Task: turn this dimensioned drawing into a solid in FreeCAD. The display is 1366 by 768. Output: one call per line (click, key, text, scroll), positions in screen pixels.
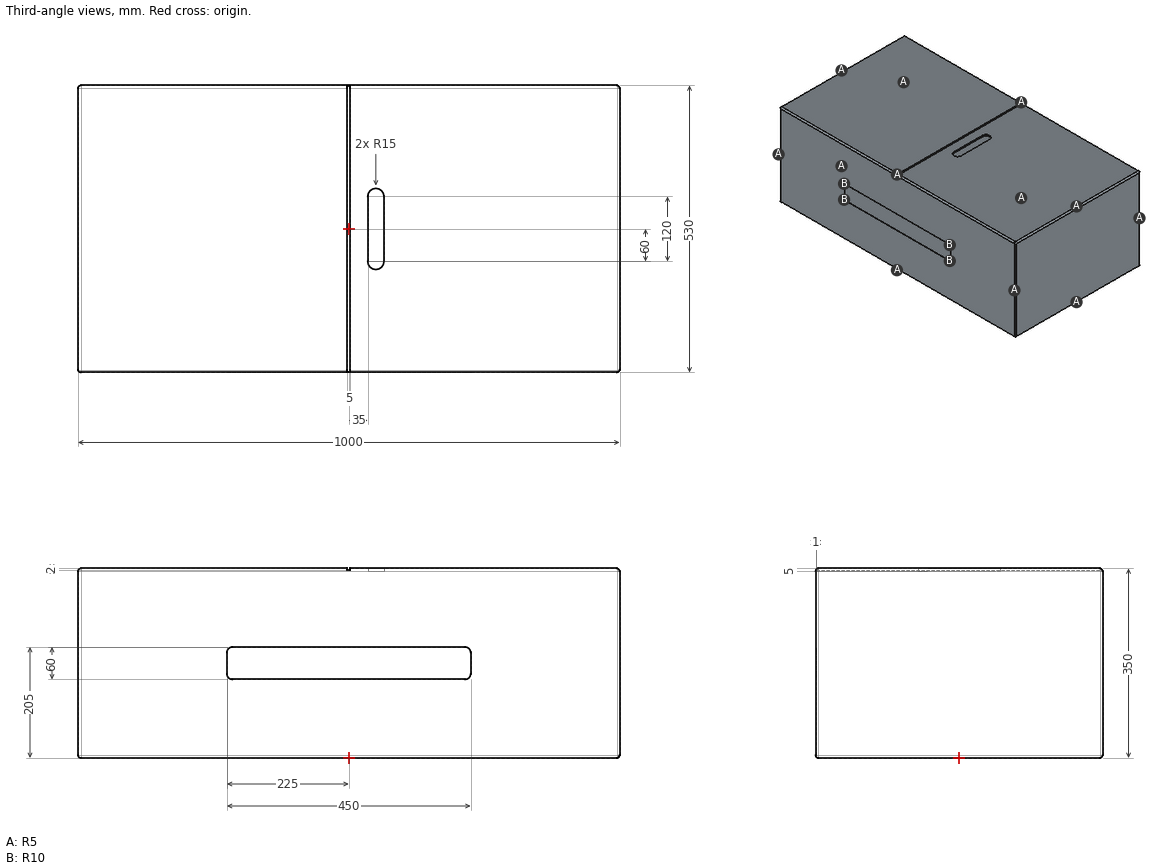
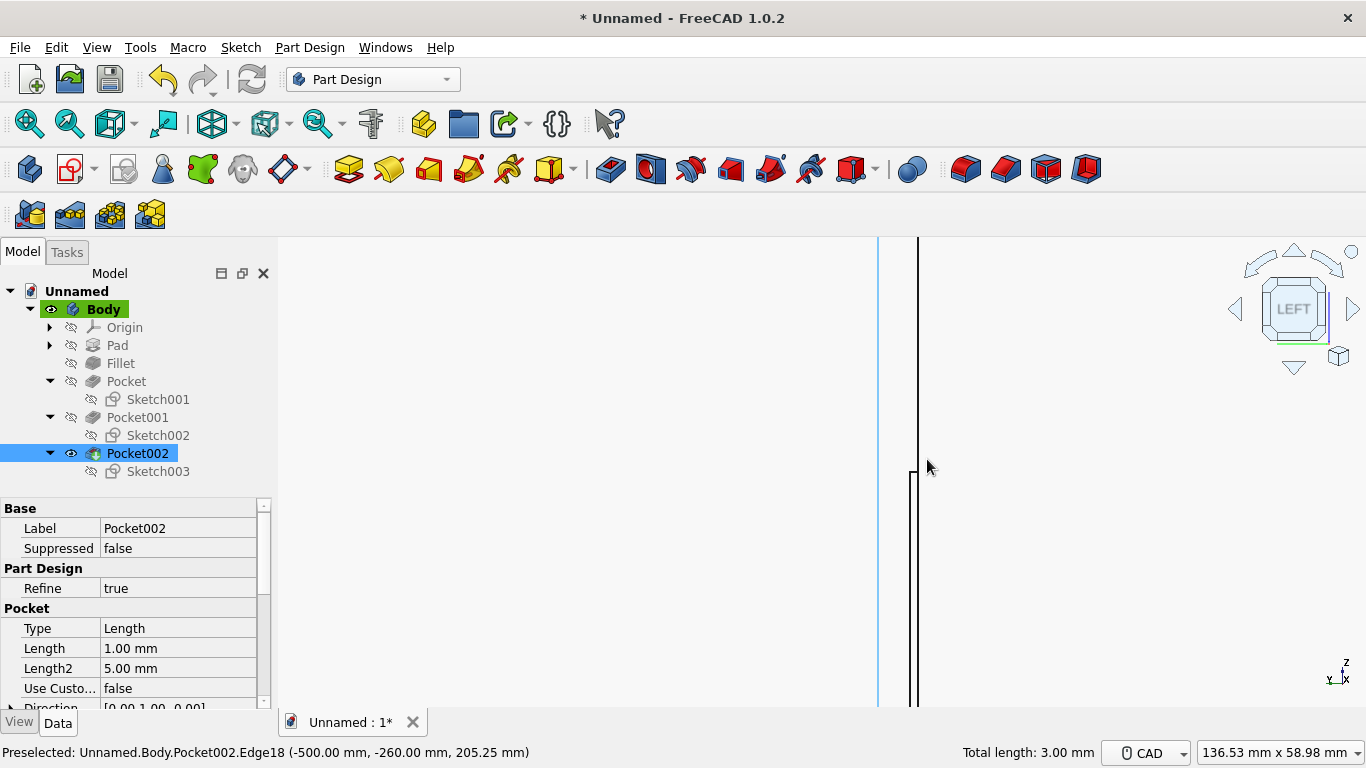
scroll(914, 471, up, 9)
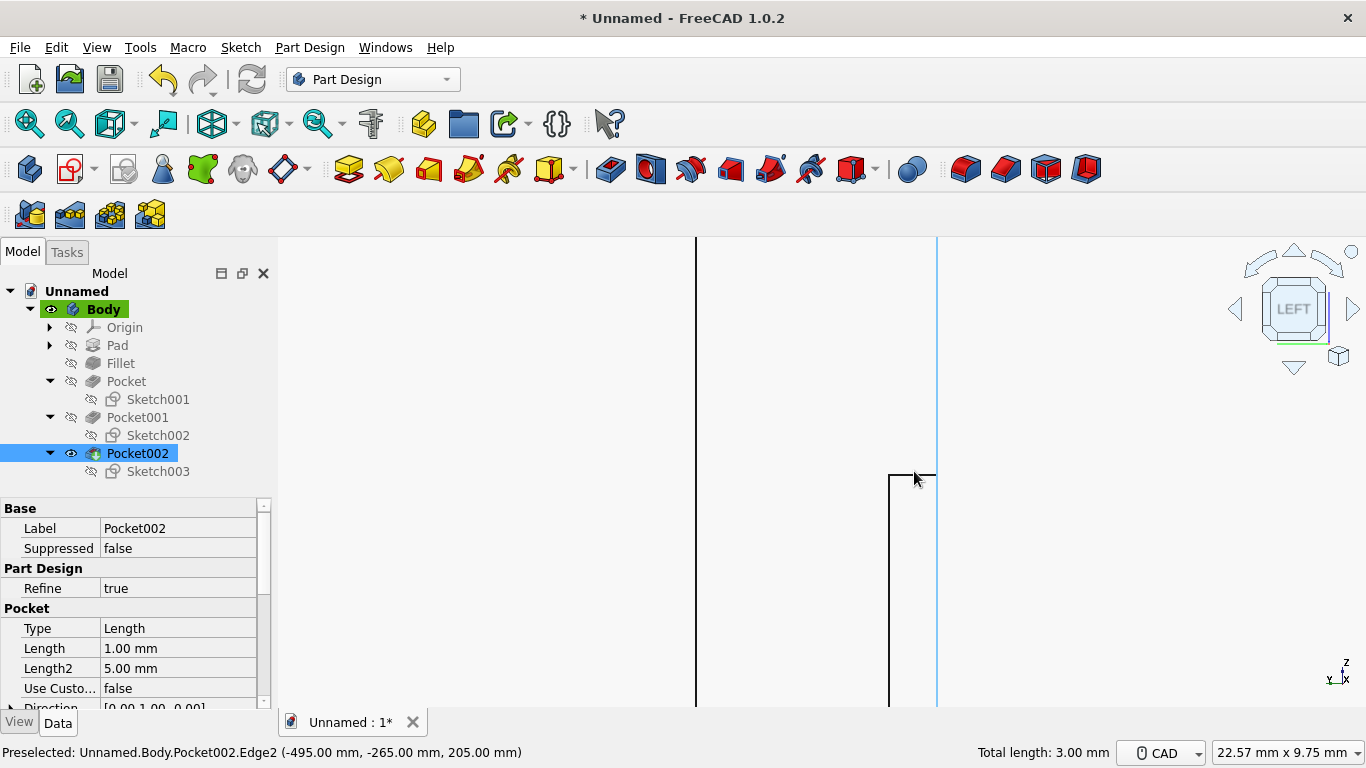
click(913, 474, ctrl)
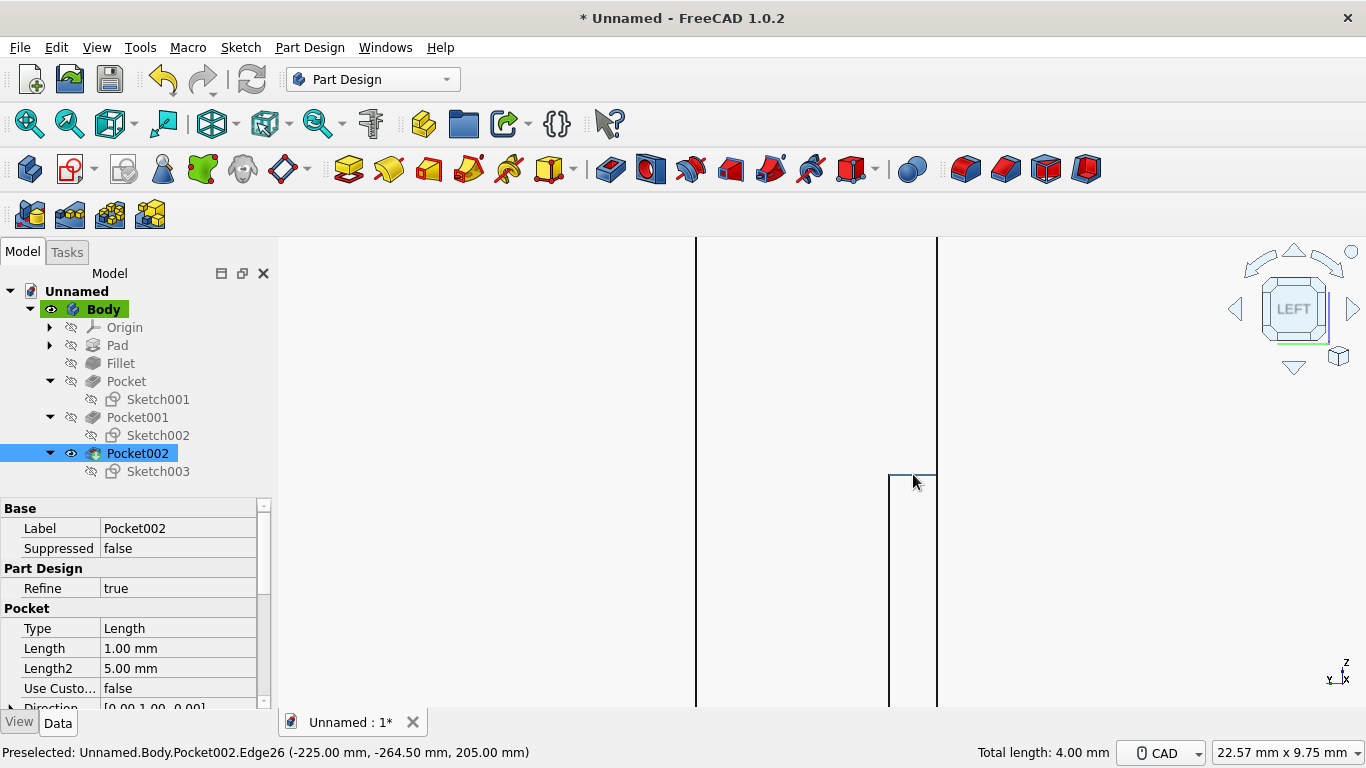
key(v)
key(1)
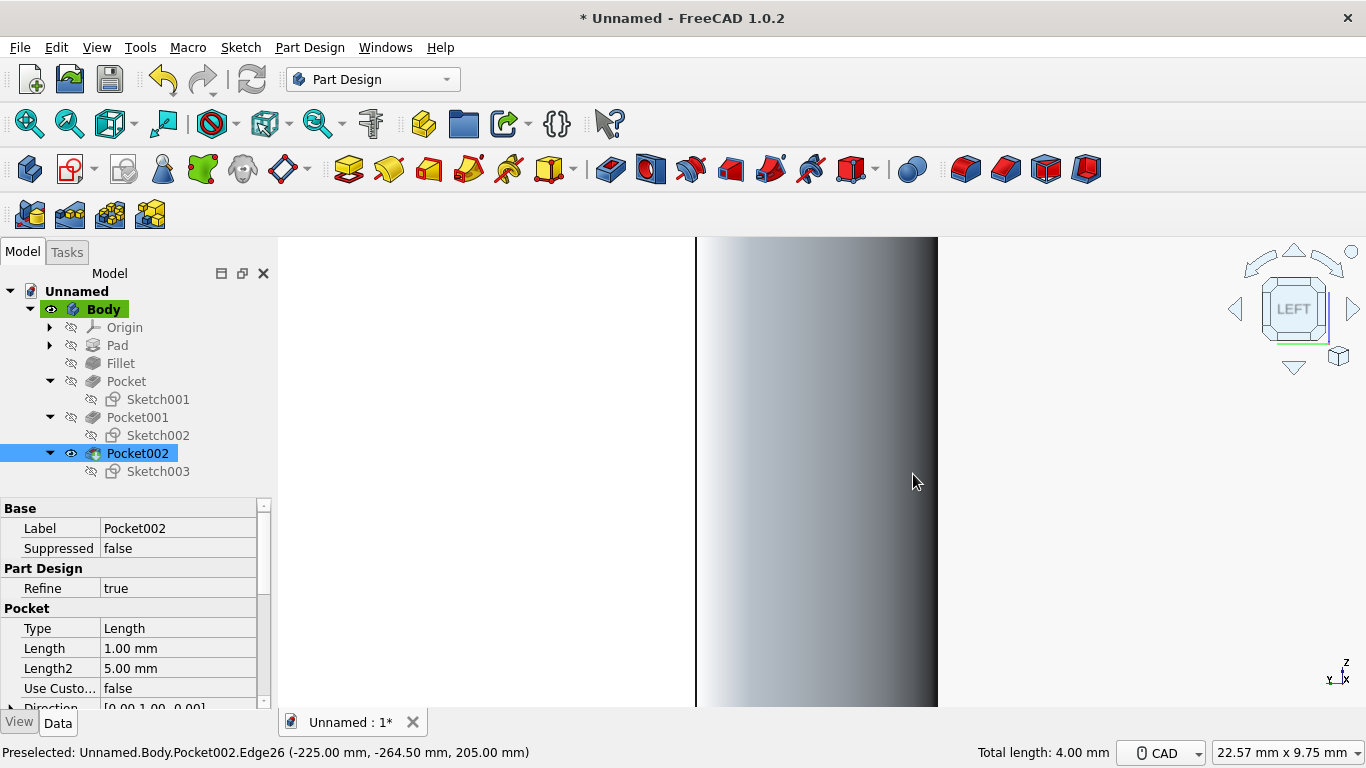
click(966, 170)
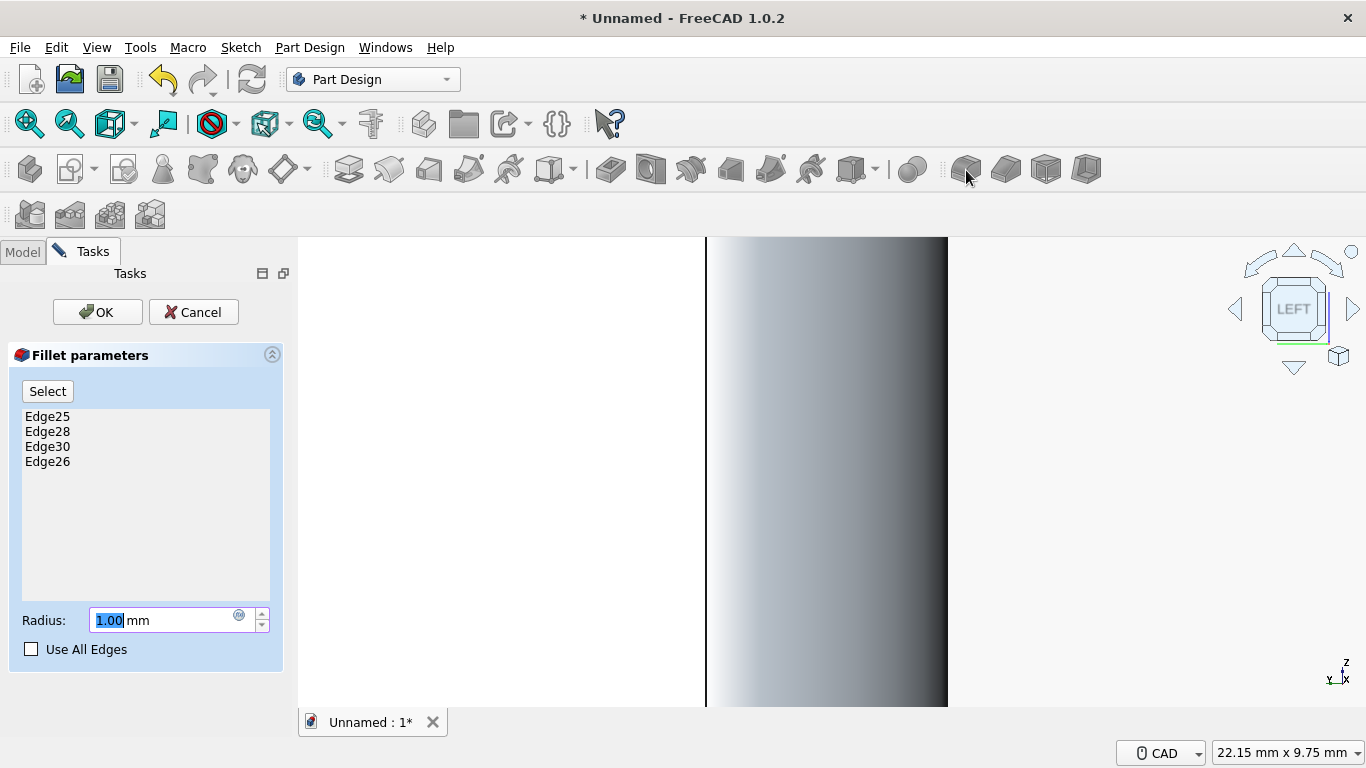
text(10)
key(Tab)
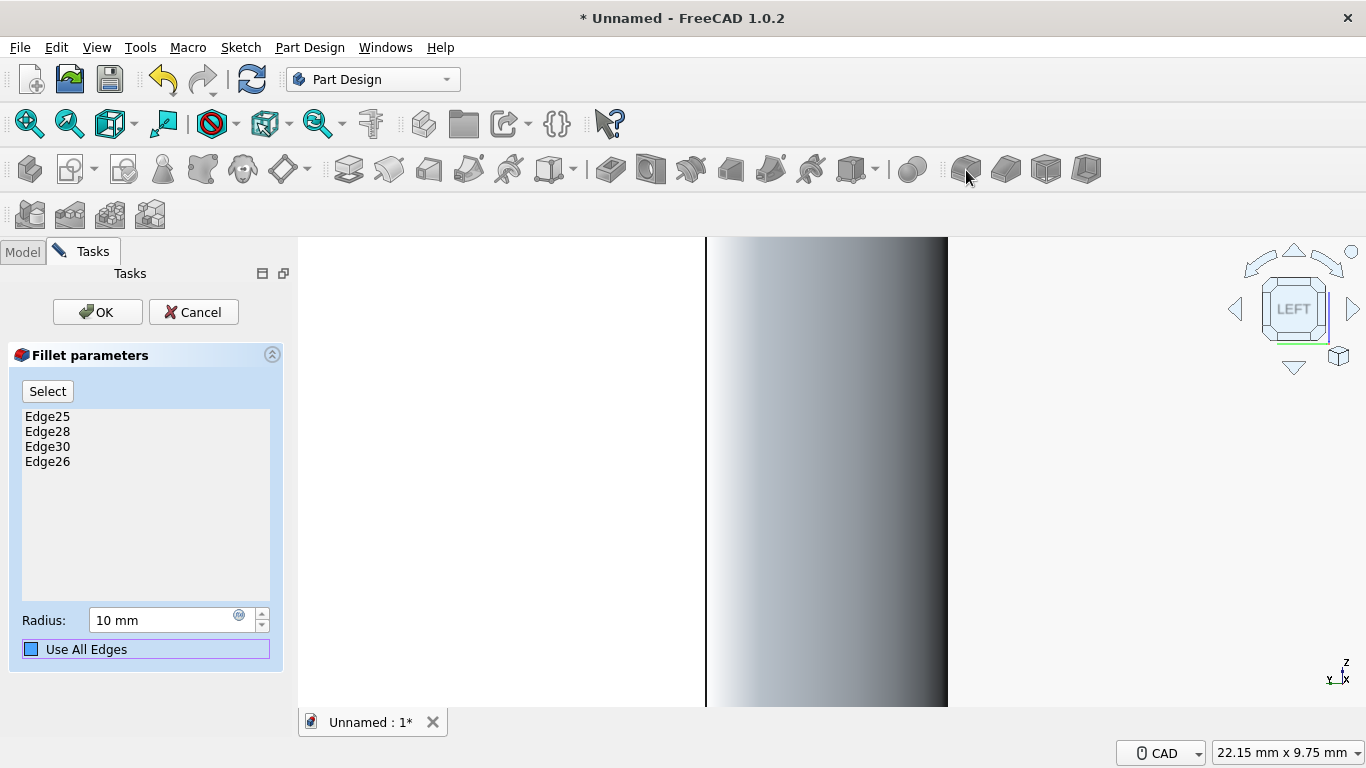
click(98, 312)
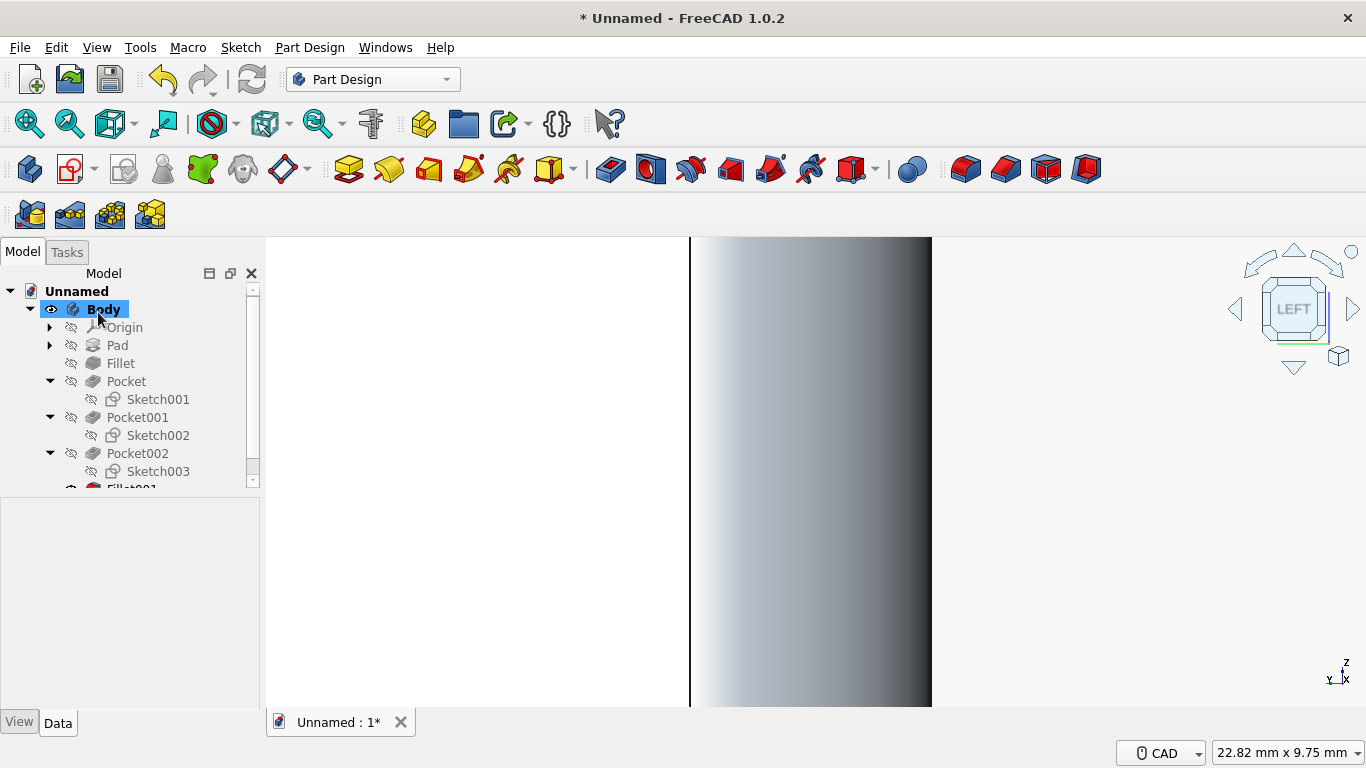
key(0)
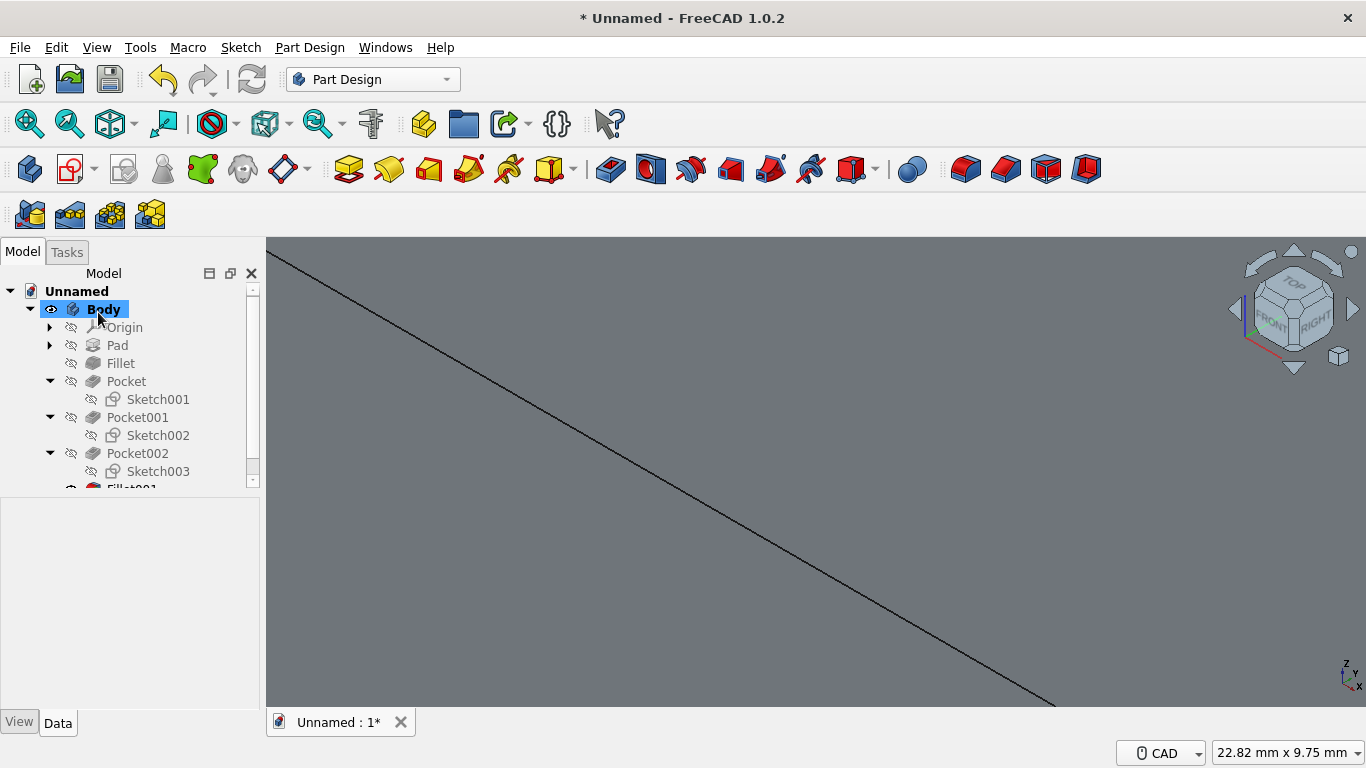
click(30, 124)